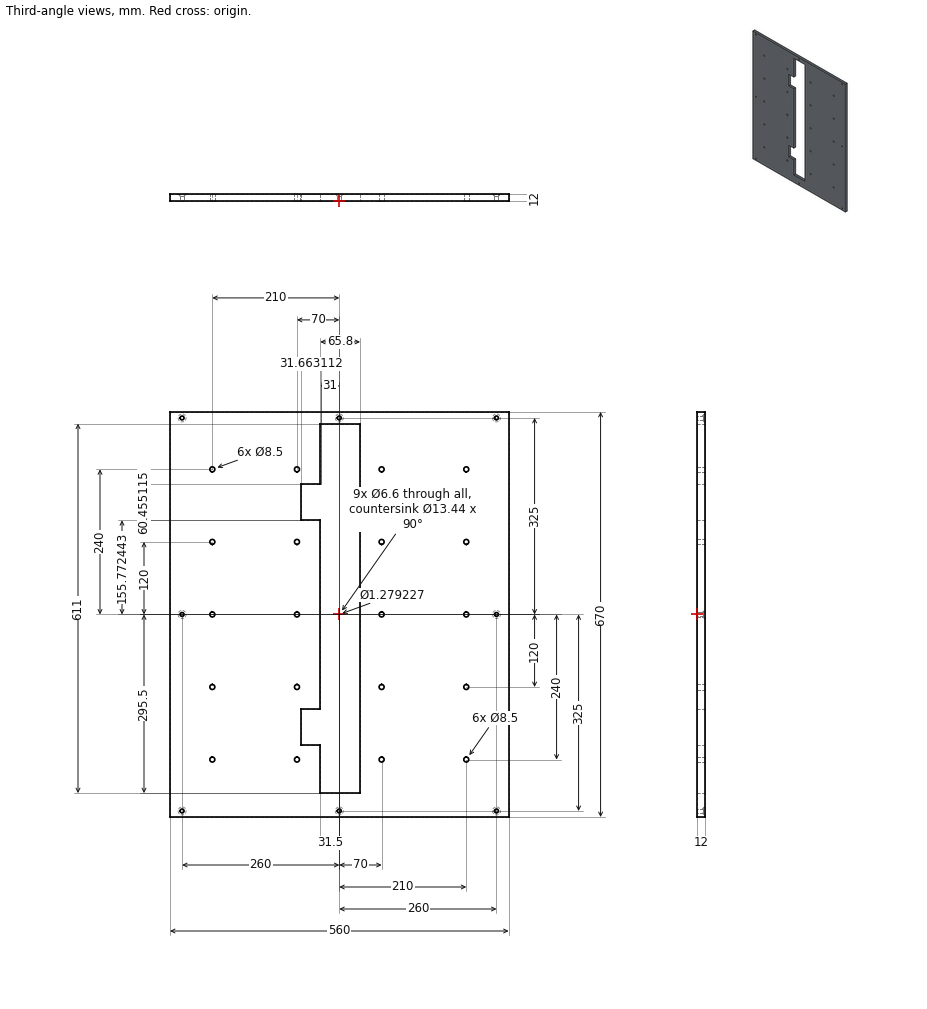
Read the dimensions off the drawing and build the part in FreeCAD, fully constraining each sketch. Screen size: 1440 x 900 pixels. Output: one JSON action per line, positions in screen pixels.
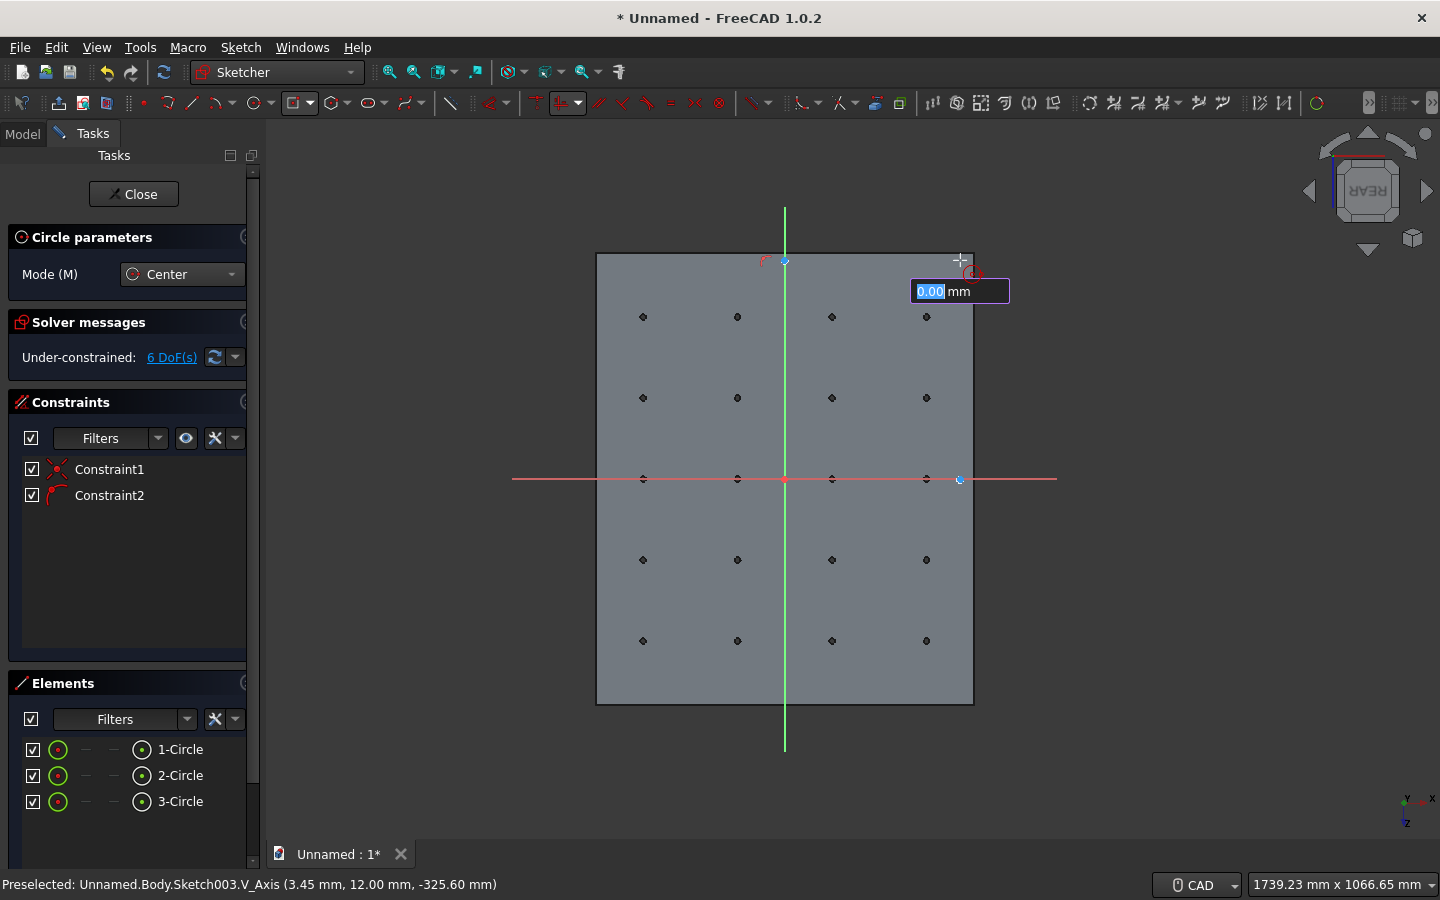
{"action": "scroll", "coordinate": [962, 258], "scroll_direction": "up", "scroll_amount": 10}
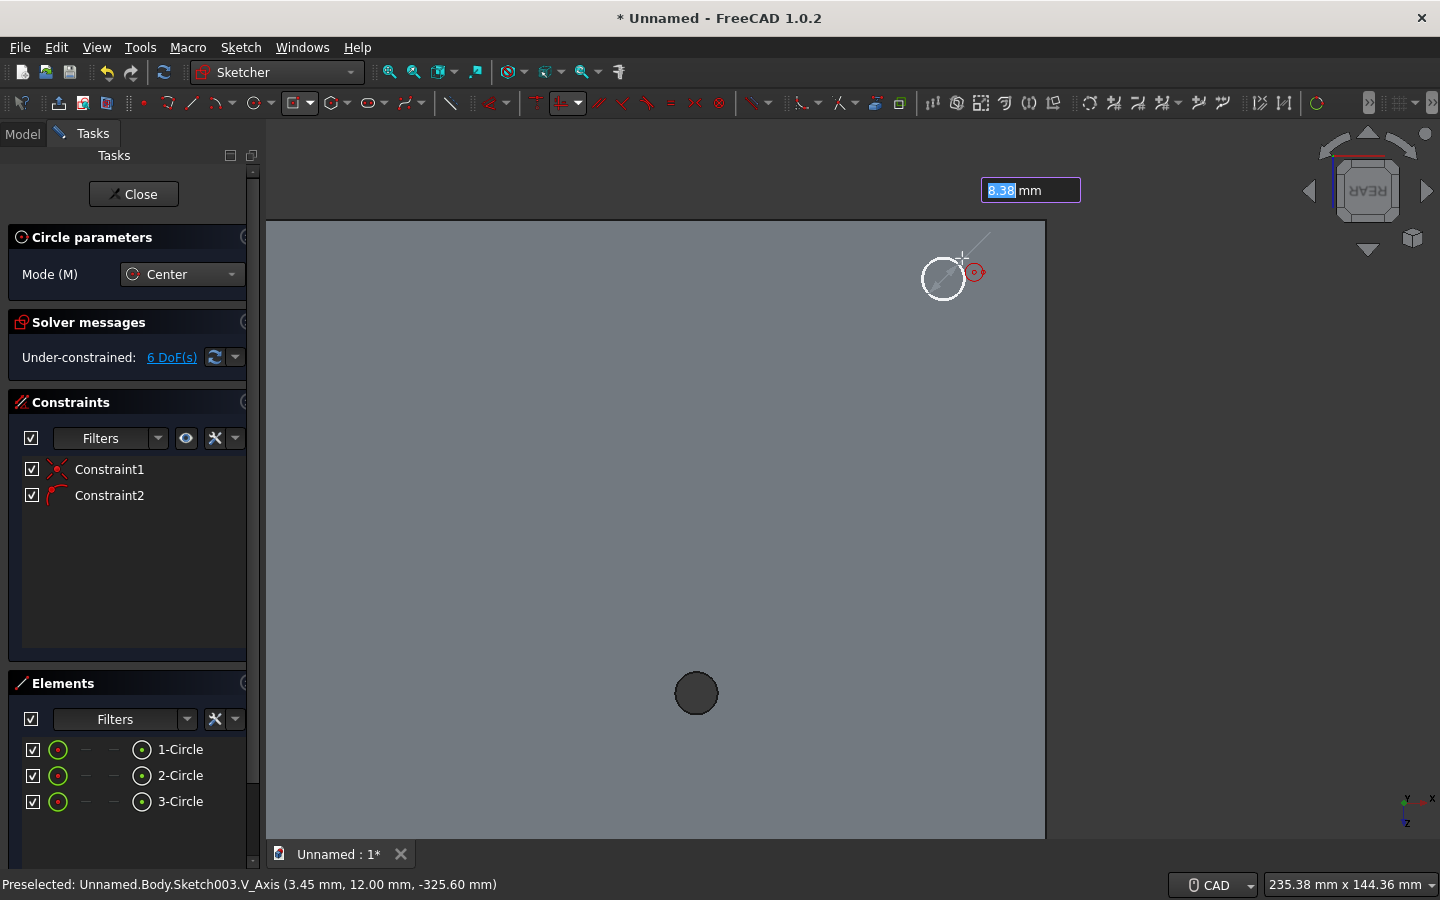
{"action": "left_click", "coordinate": [958, 258]}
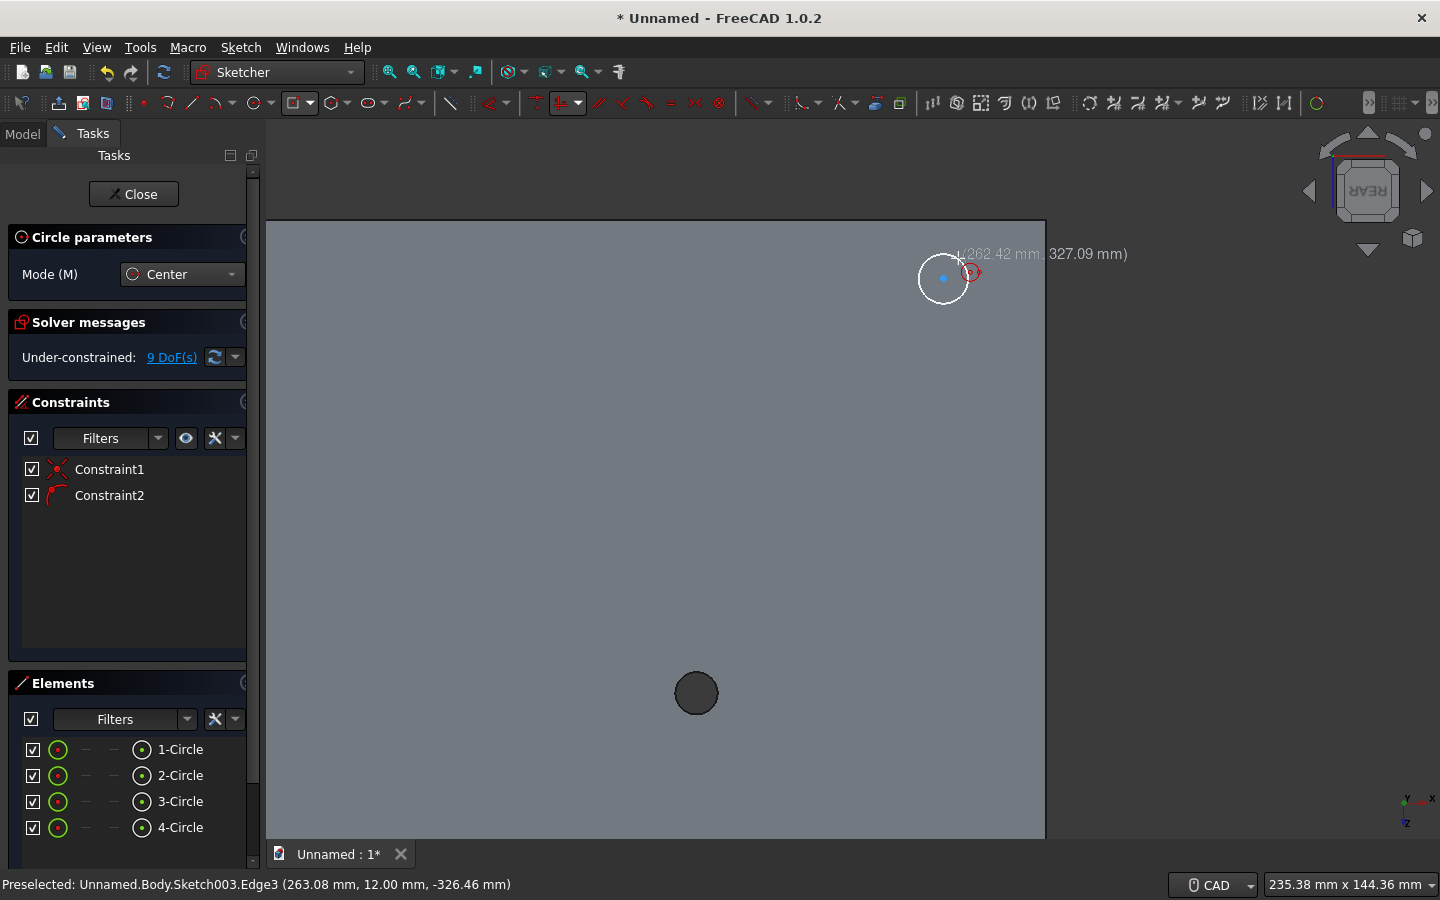
{"action": "scroll", "coordinate": [962, 258], "scroll_direction": "down", "scroll_amount": 10}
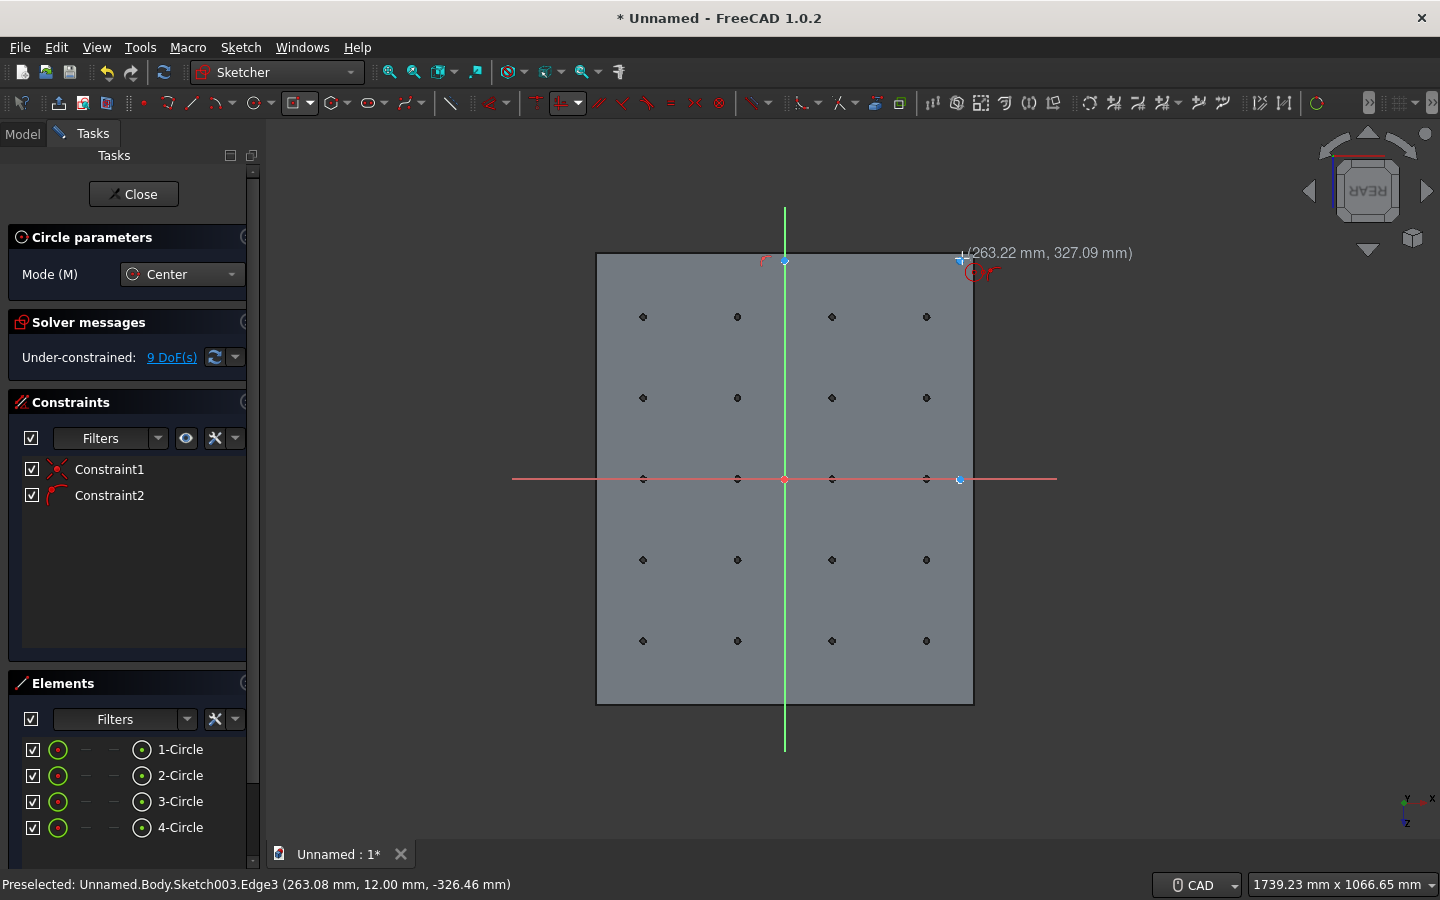
{"action": "scroll", "coordinate": [785, 698], "scroll_direction": "up", "scroll_amount": 12}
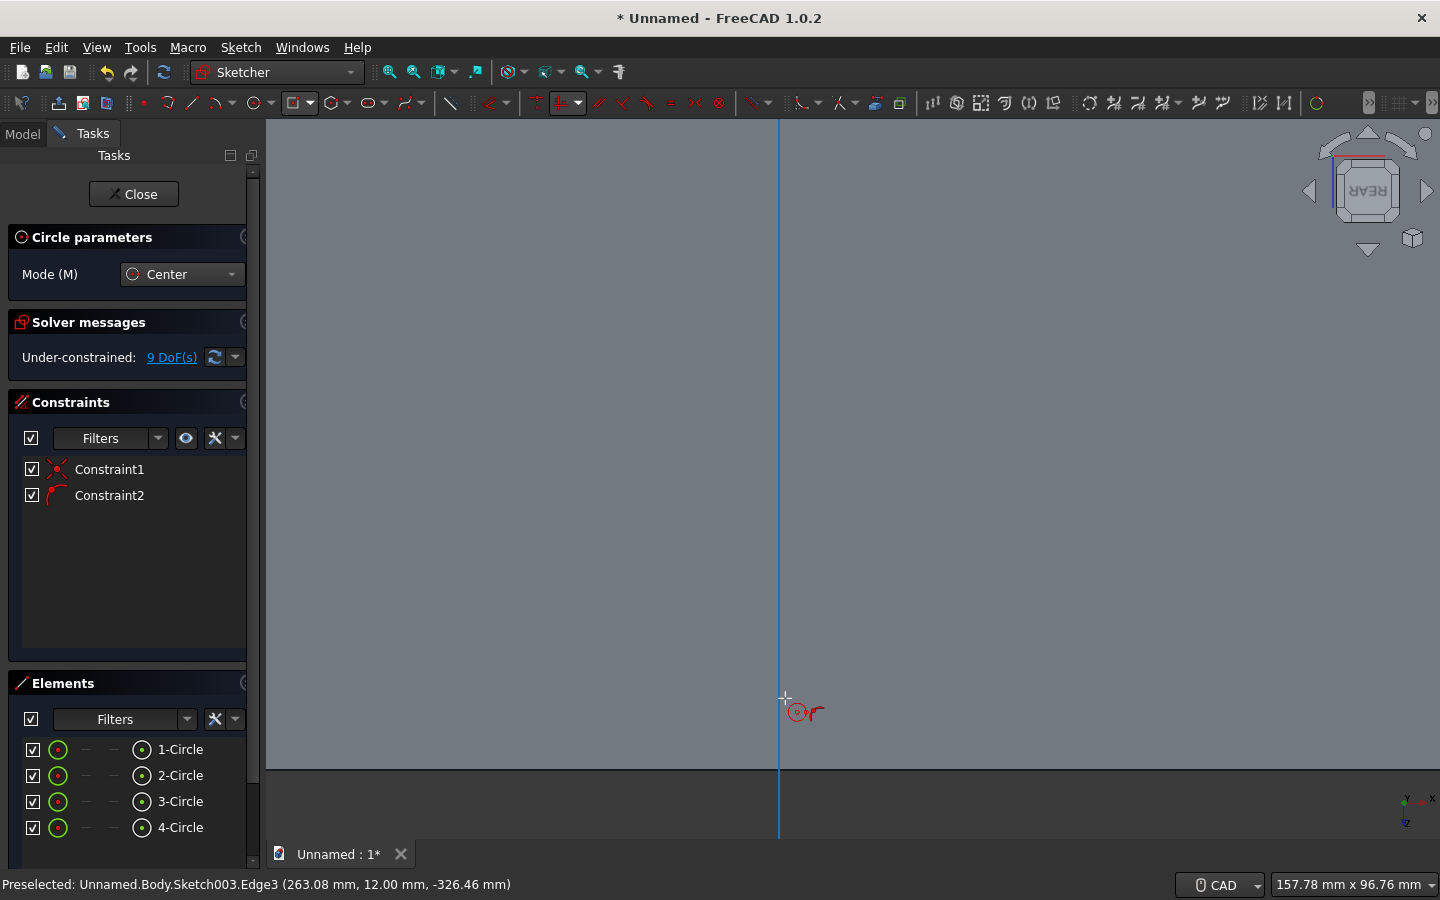
{"action": "scroll", "coordinate": [785, 699], "scroll_direction": "down", "scroll_amount": 12}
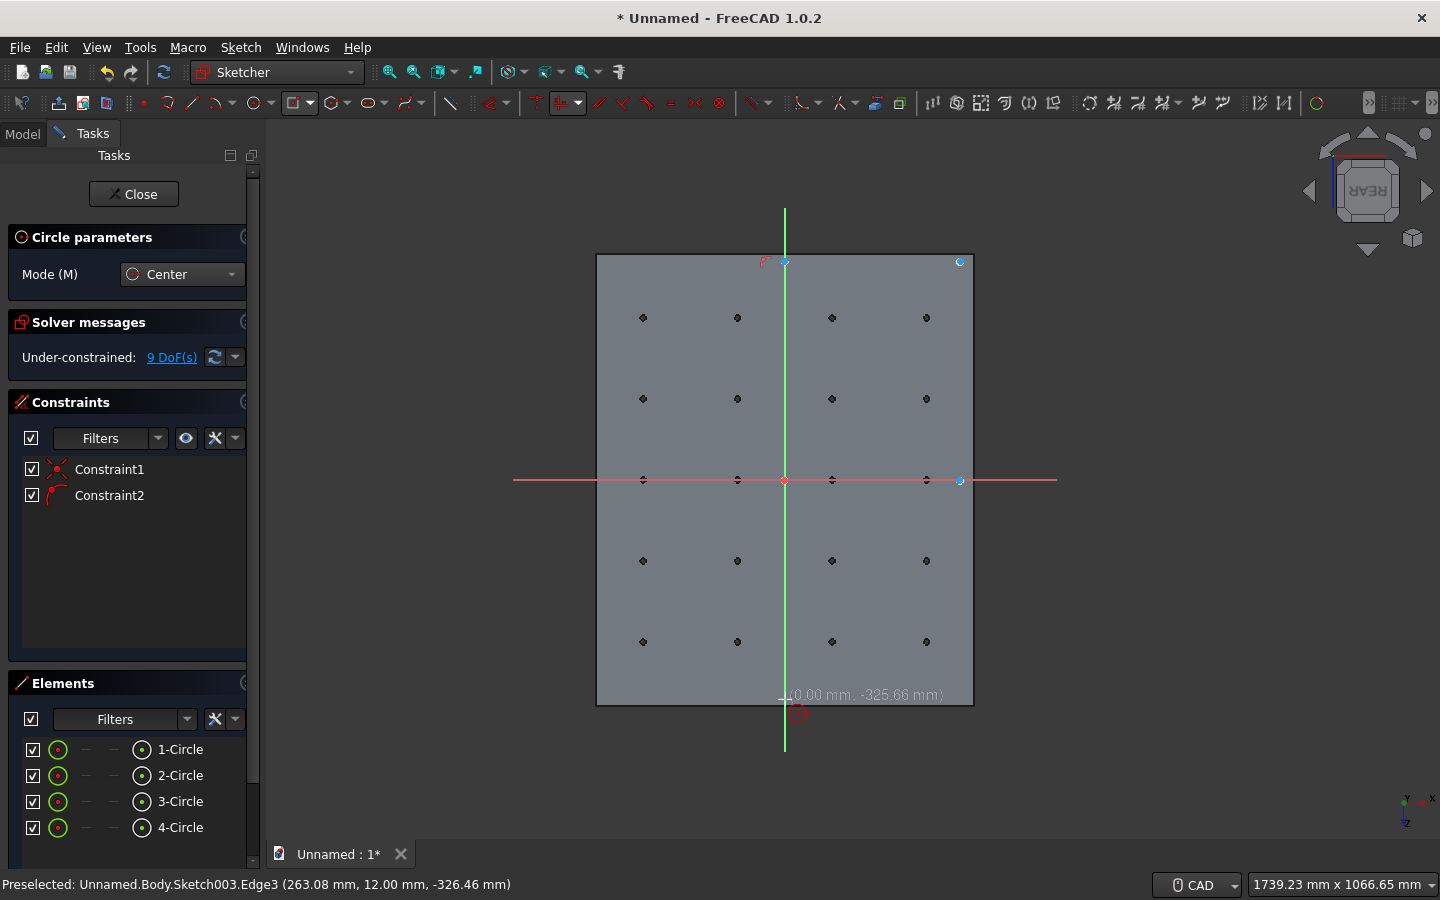
{"action": "left_click", "coordinate": [785, 699]}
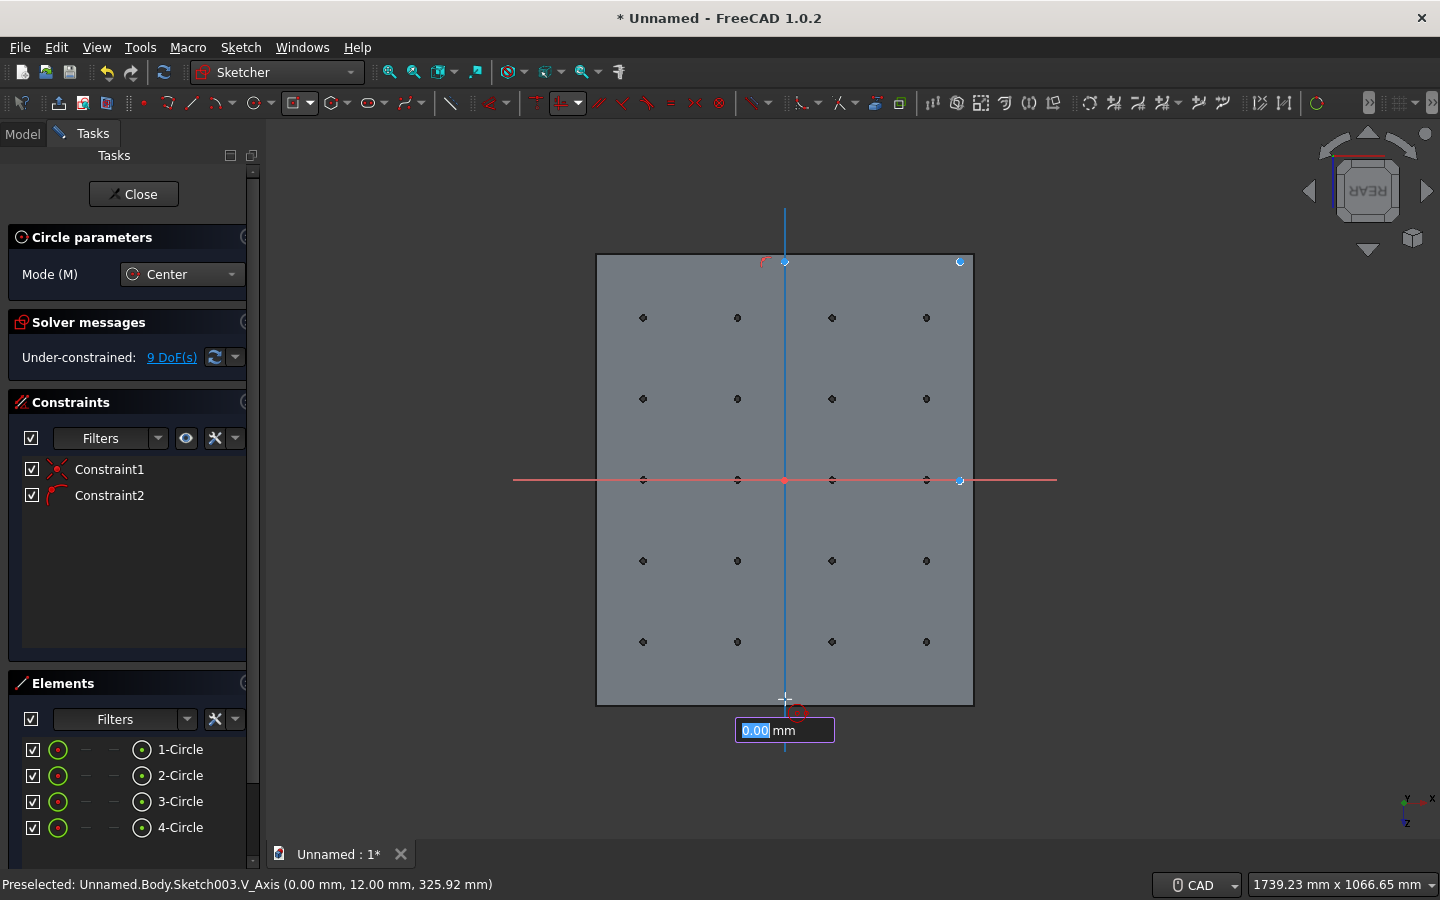
{"action": "scroll", "coordinate": [787, 699], "scroll_direction": "up", "scroll_amount": 11}